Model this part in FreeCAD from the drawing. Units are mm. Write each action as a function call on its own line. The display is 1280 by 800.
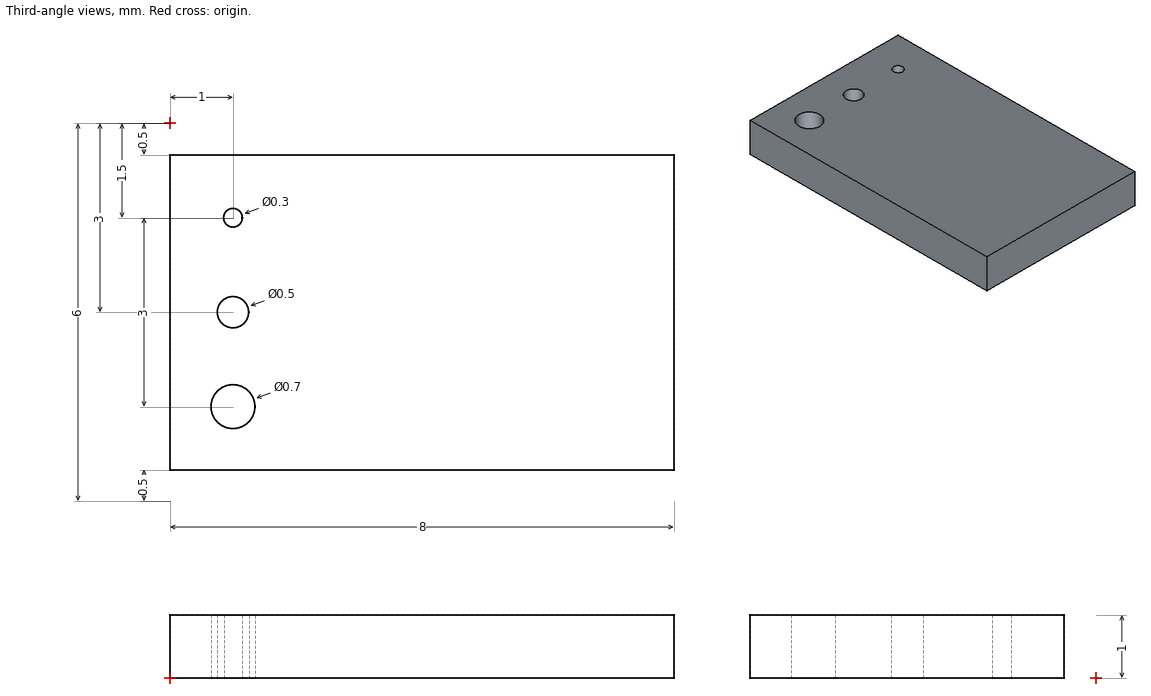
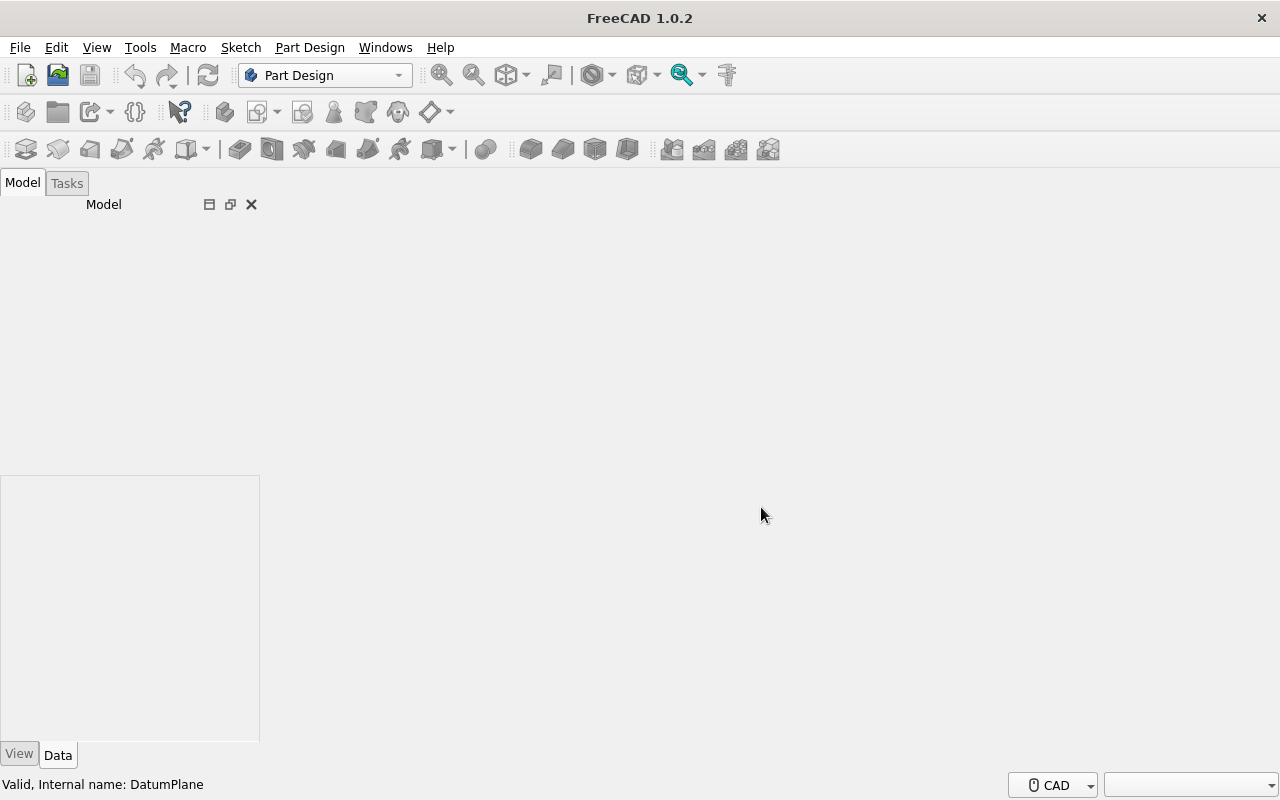
key(ctrl+n)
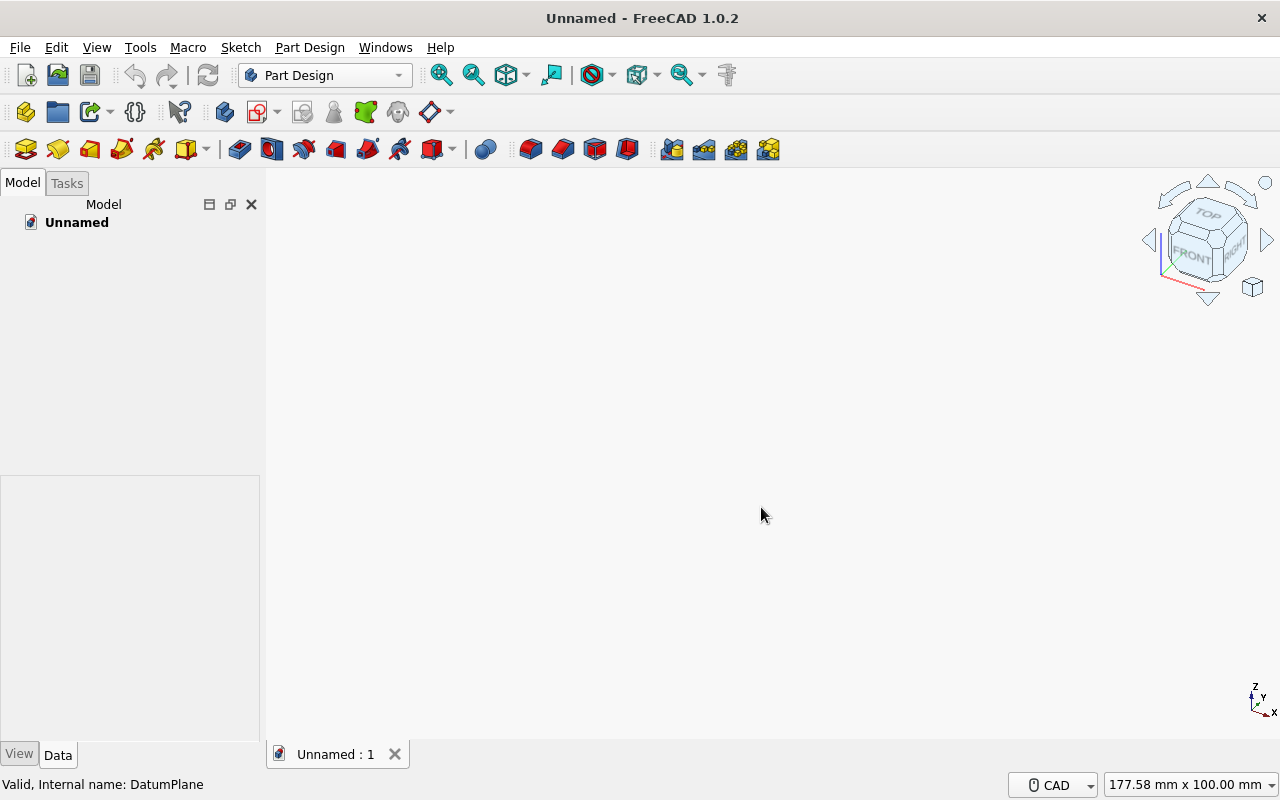
click(258, 112)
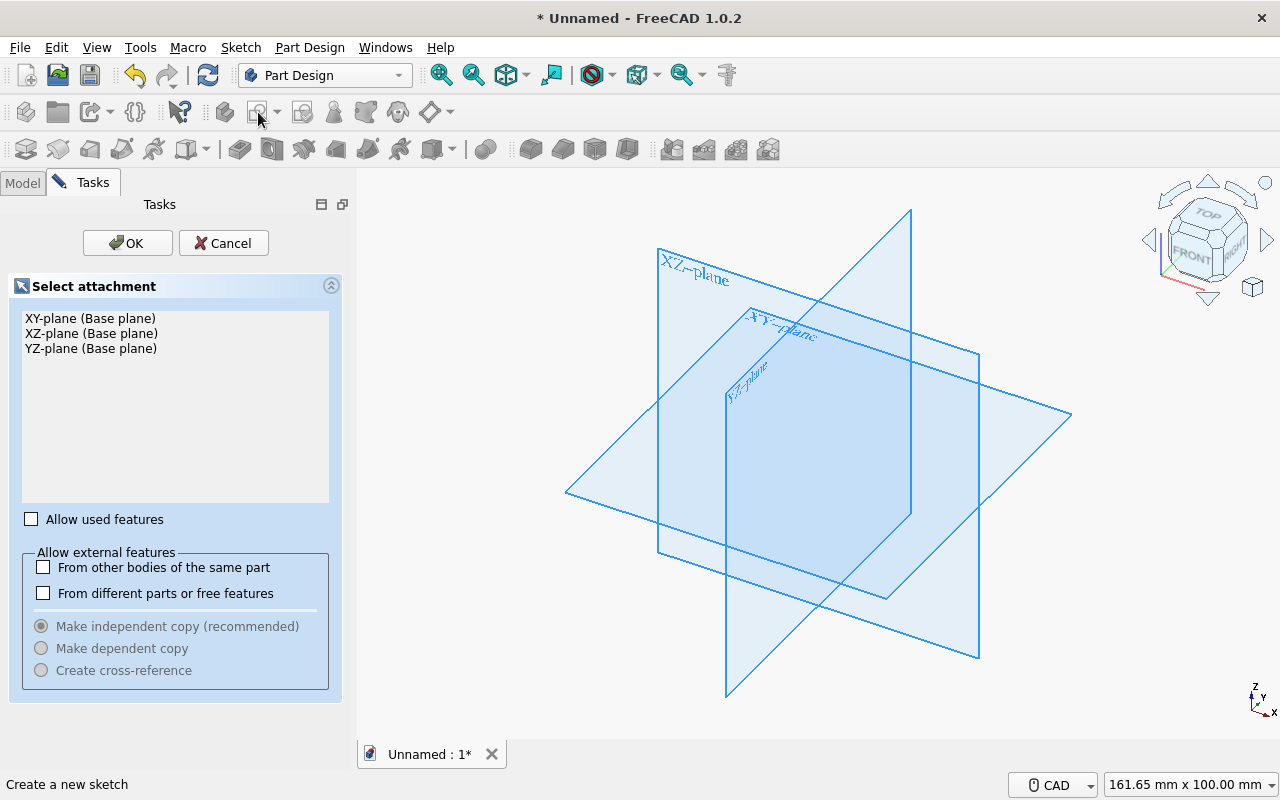
click(82, 318)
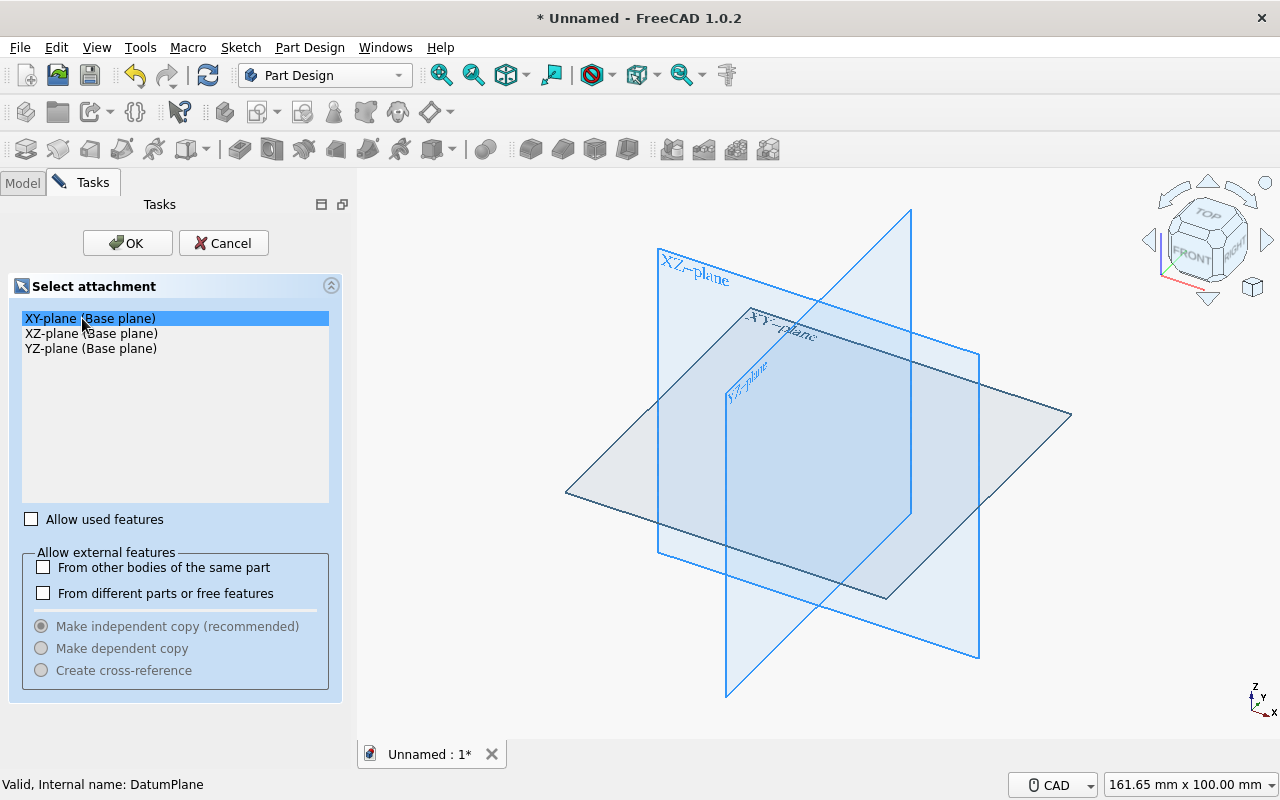
click(128, 243)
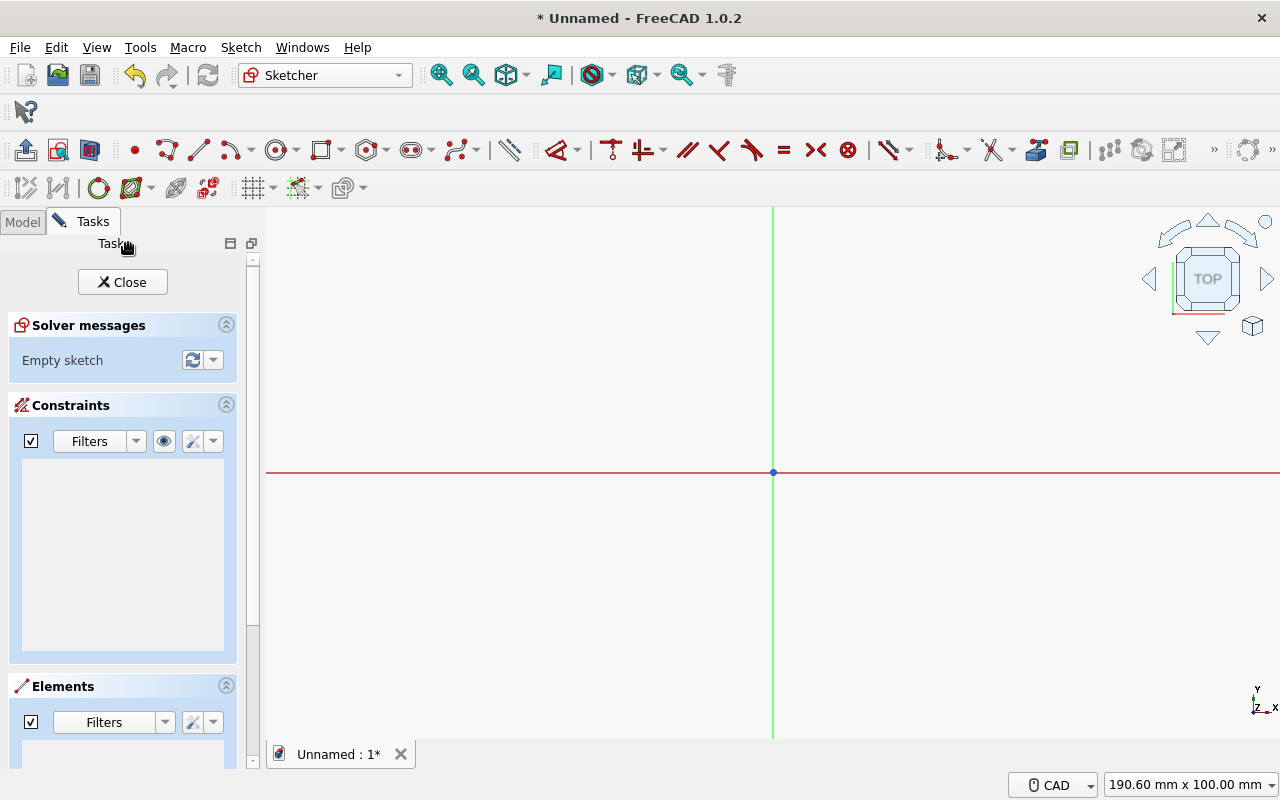
scroll(803, 491, up, 12)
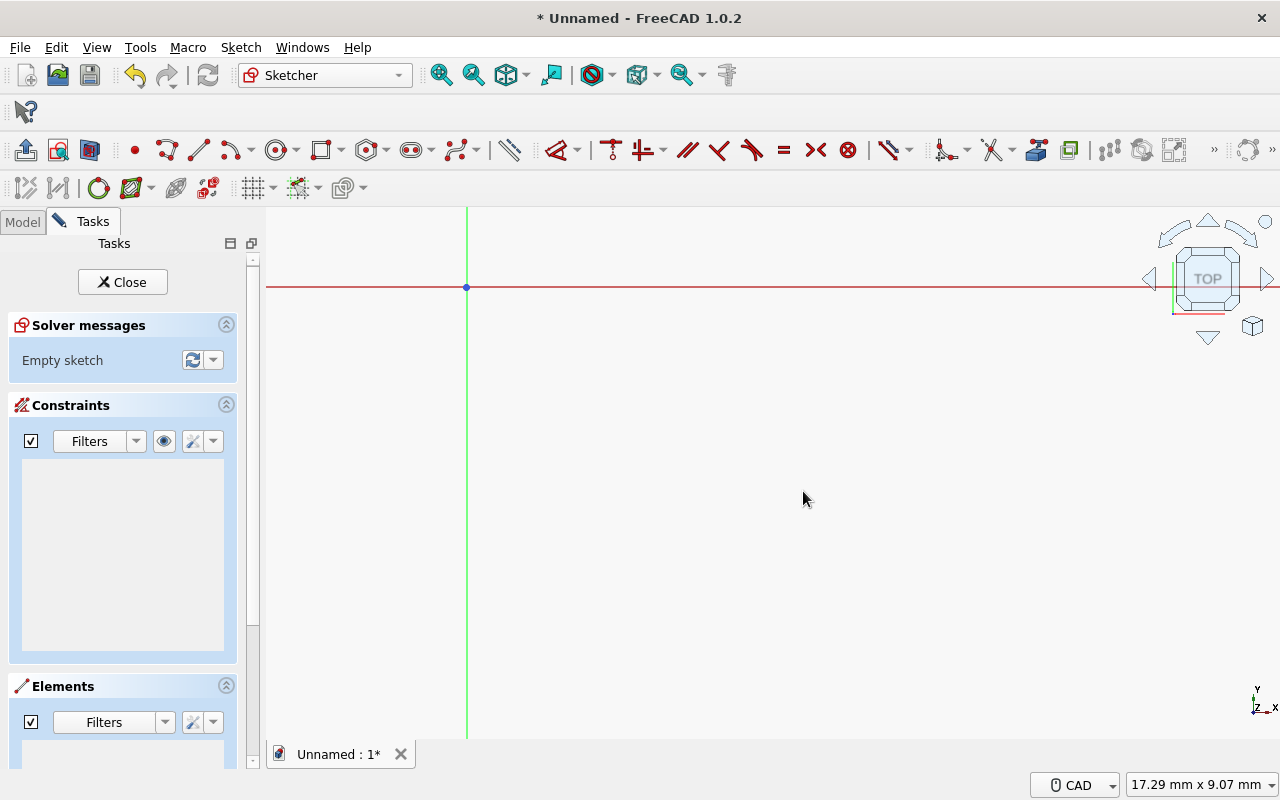
key(g)
key(r)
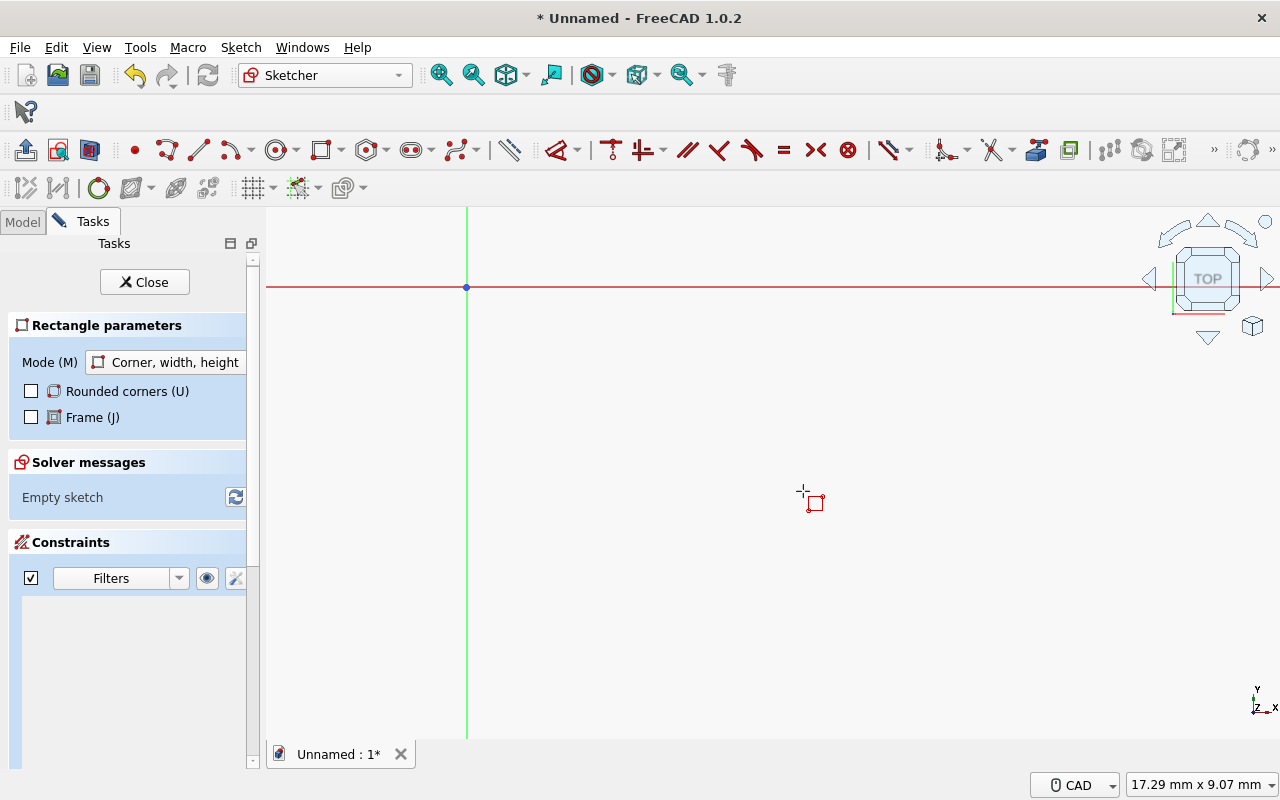
click(467, 287)
click(936, 639)
key(Escape)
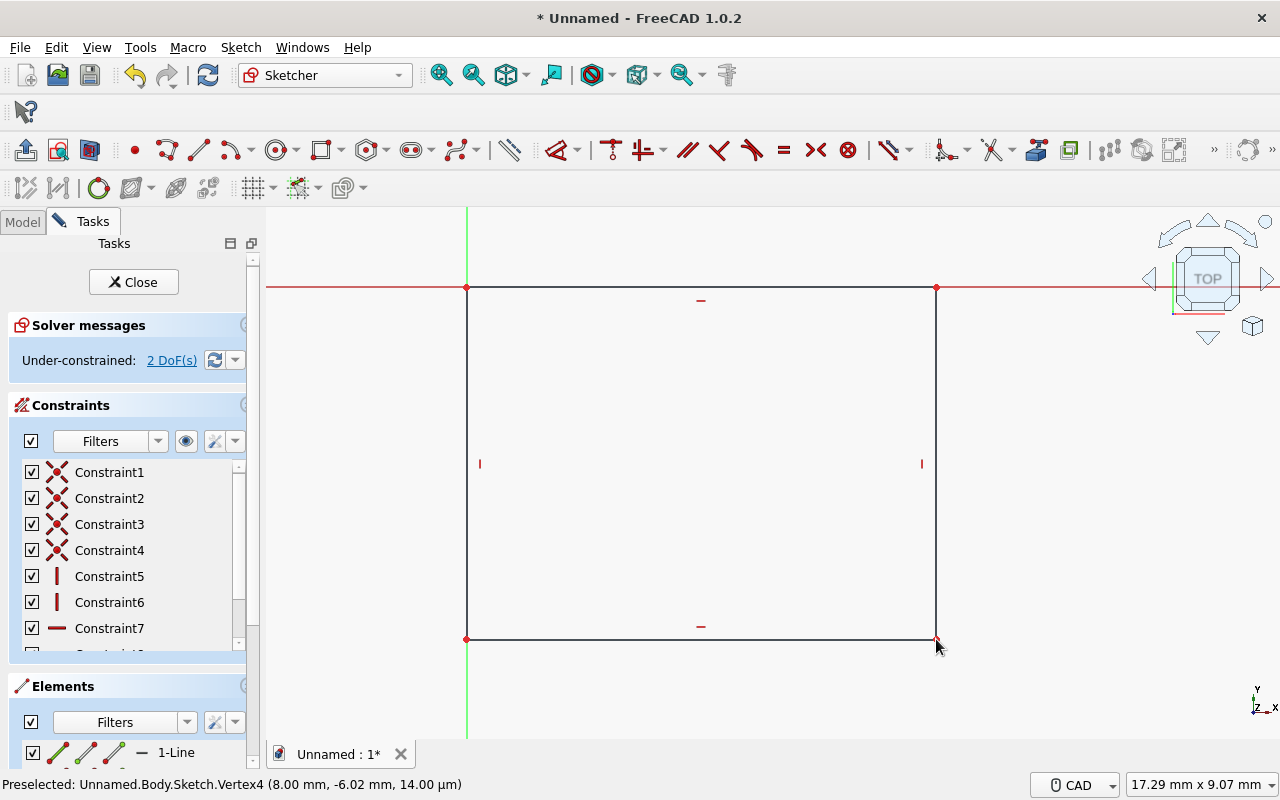
click(467, 393)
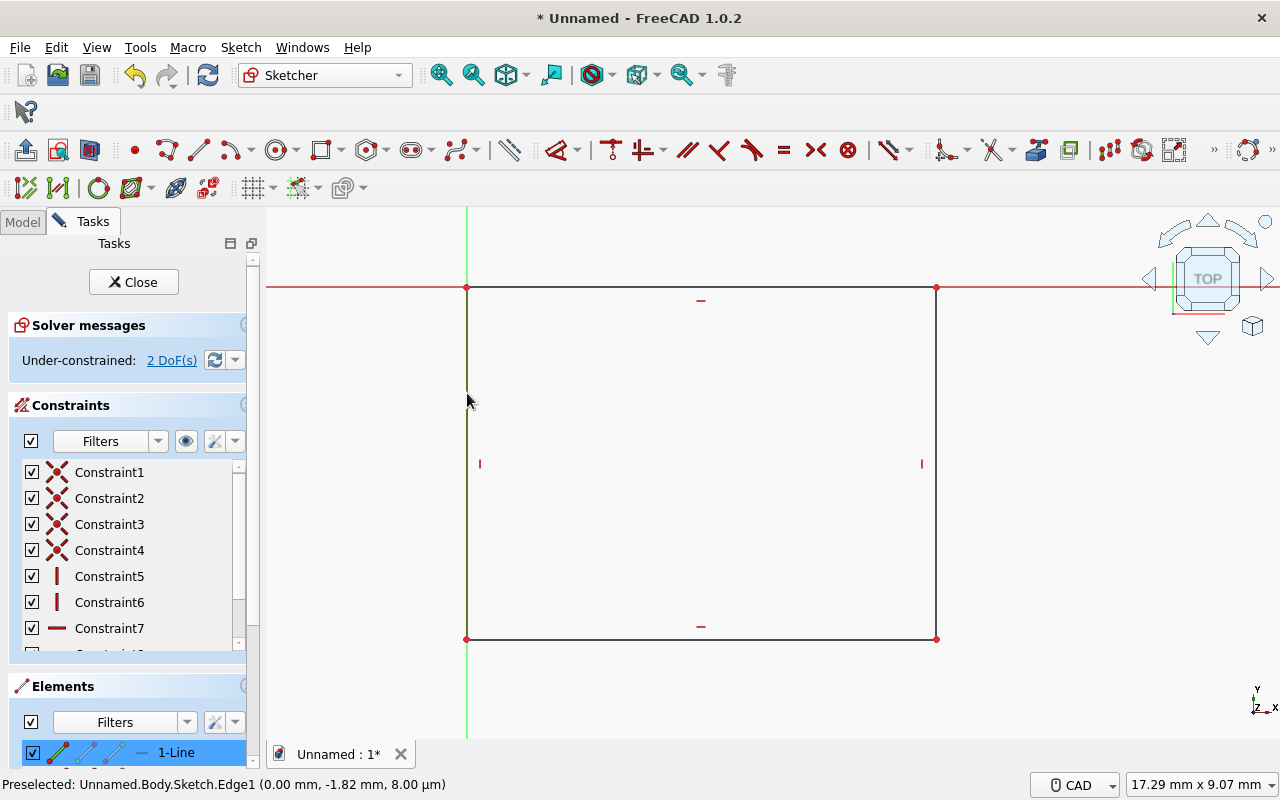
key(i)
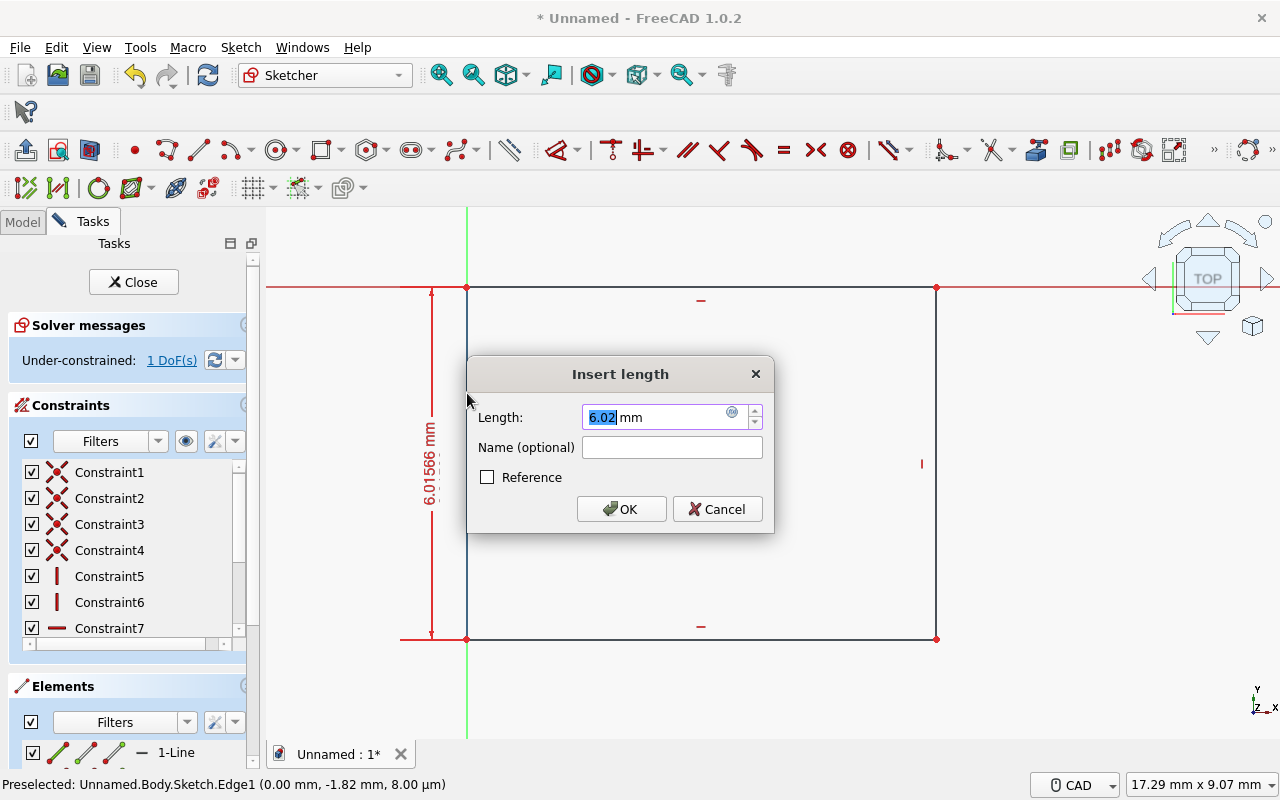
text(6)
key(Return)